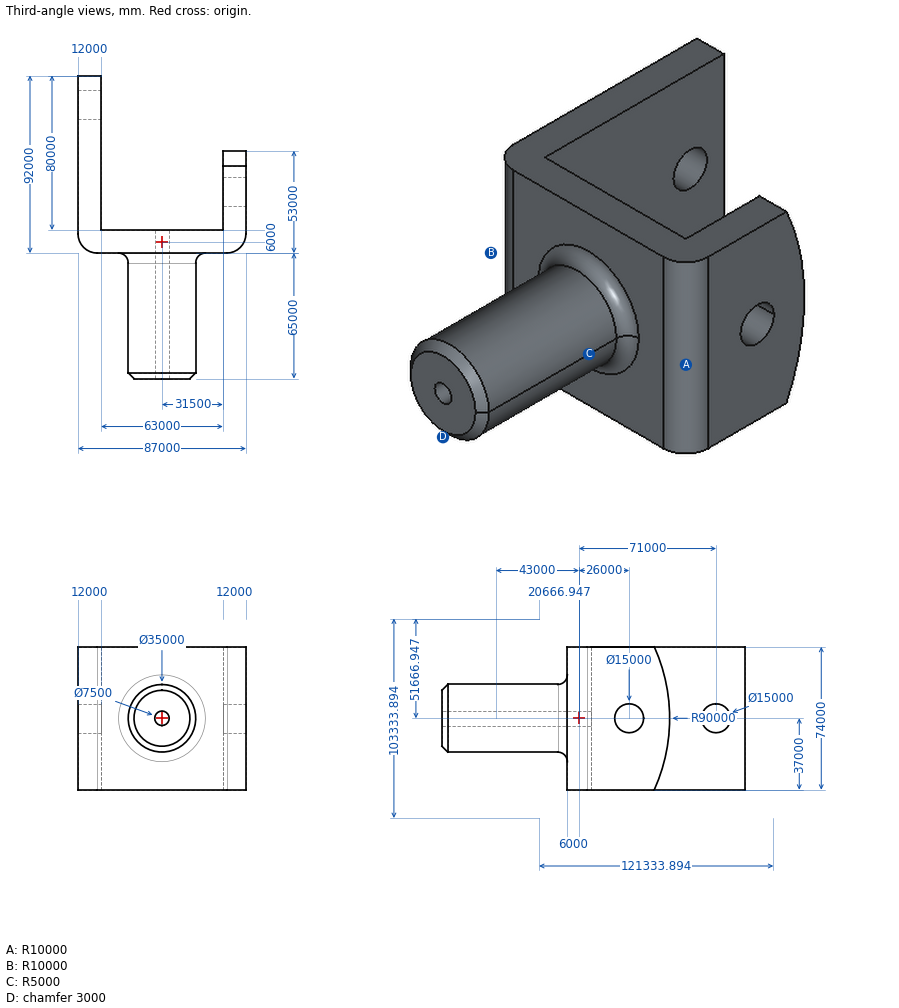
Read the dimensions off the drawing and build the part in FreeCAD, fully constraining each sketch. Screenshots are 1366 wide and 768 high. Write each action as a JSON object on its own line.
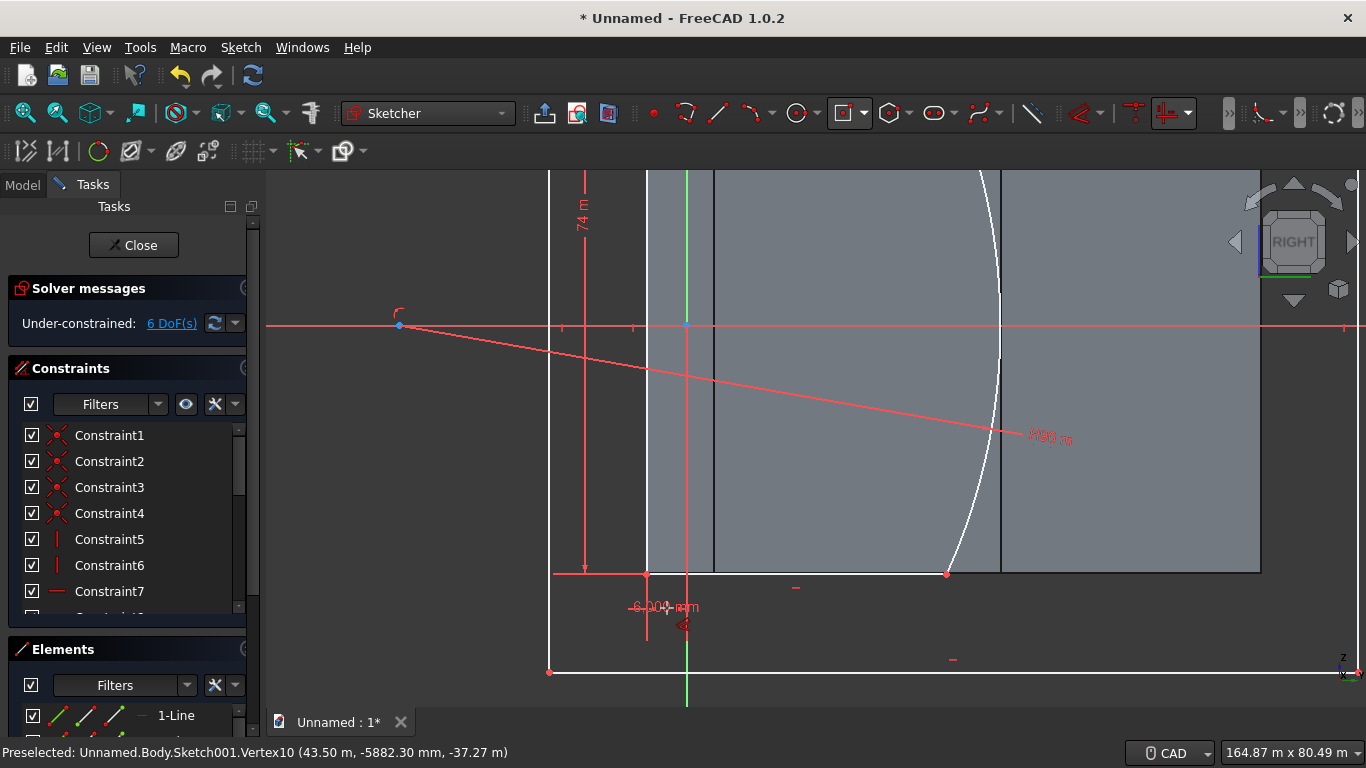
{"action": "left_click", "coordinate": [947, 574]}
{"action": "left_click", "coordinate": [981, 393]}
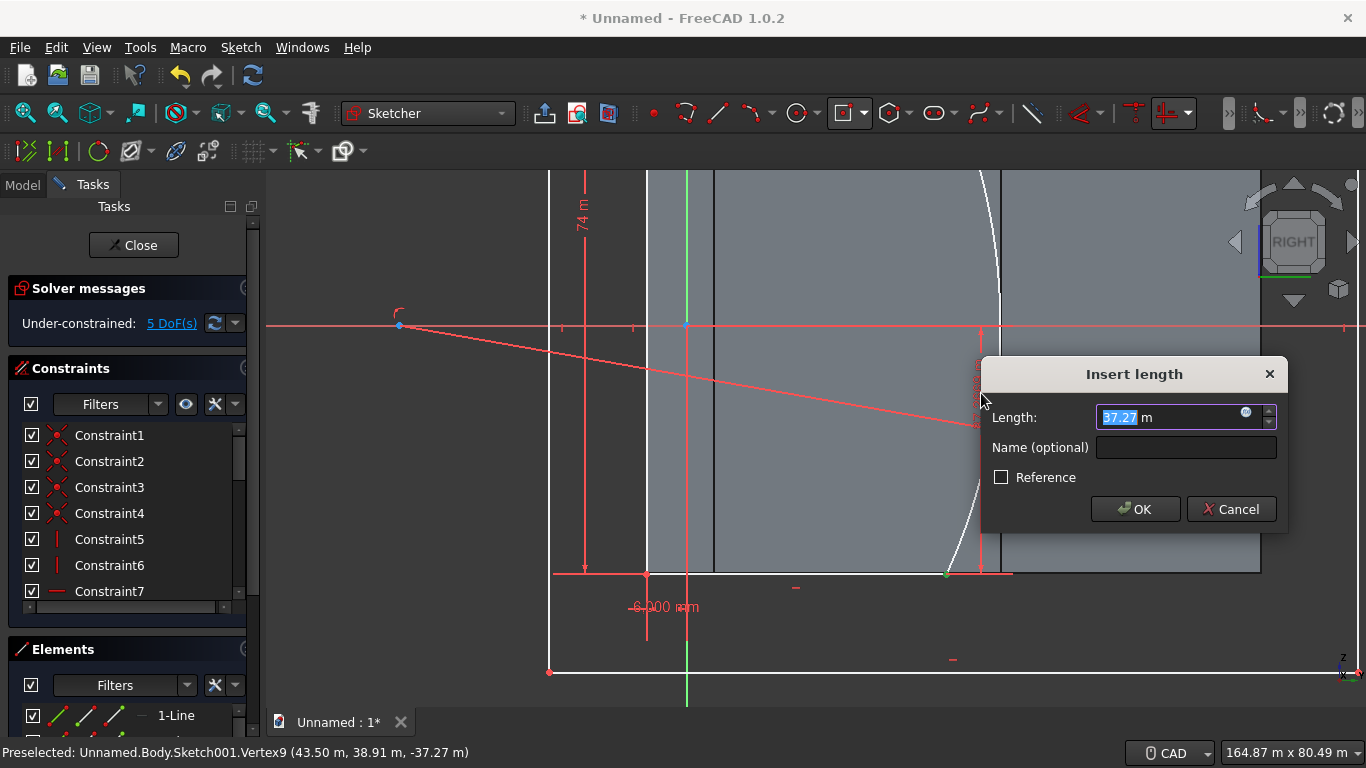
{"action": "key", "text": "ctrl+a"}
{"action": "type", "text": "37000 mm"}
{"action": "key", "text": "Return"}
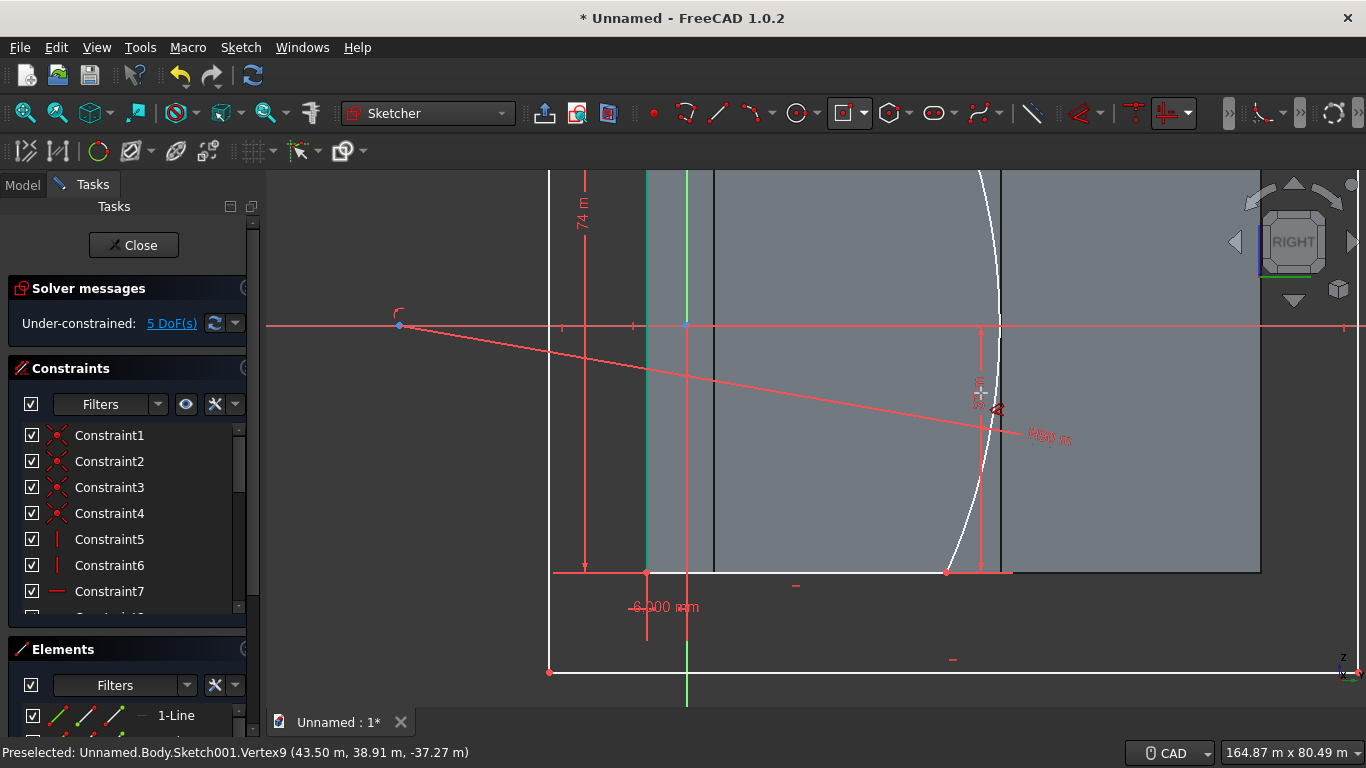
{"action": "left_click", "coordinate": [399, 326]}
{"action": "left_click", "coordinate": [477, 360]}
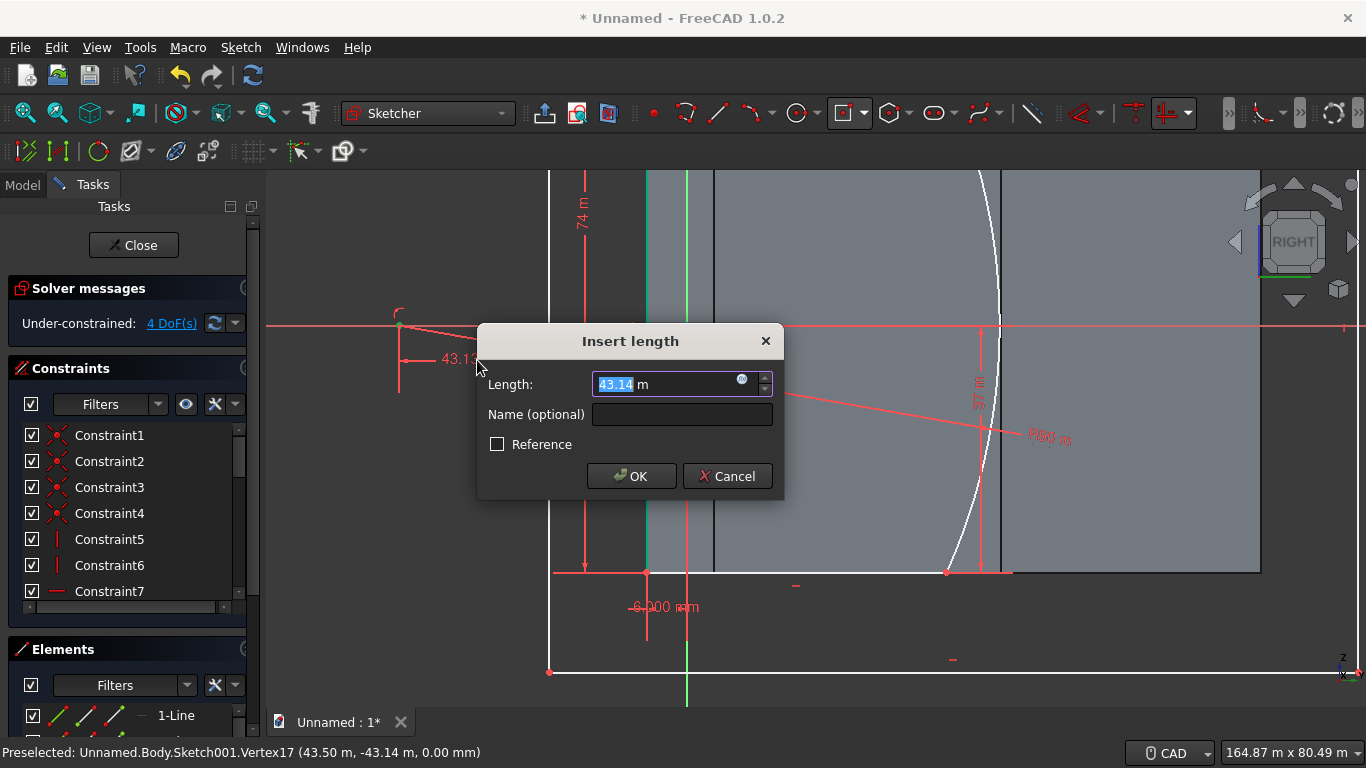
{"action": "key", "text": "ctrl+a"}
{"action": "type", "text": "43000 mm"}
{"action": "key", "text": "Return"}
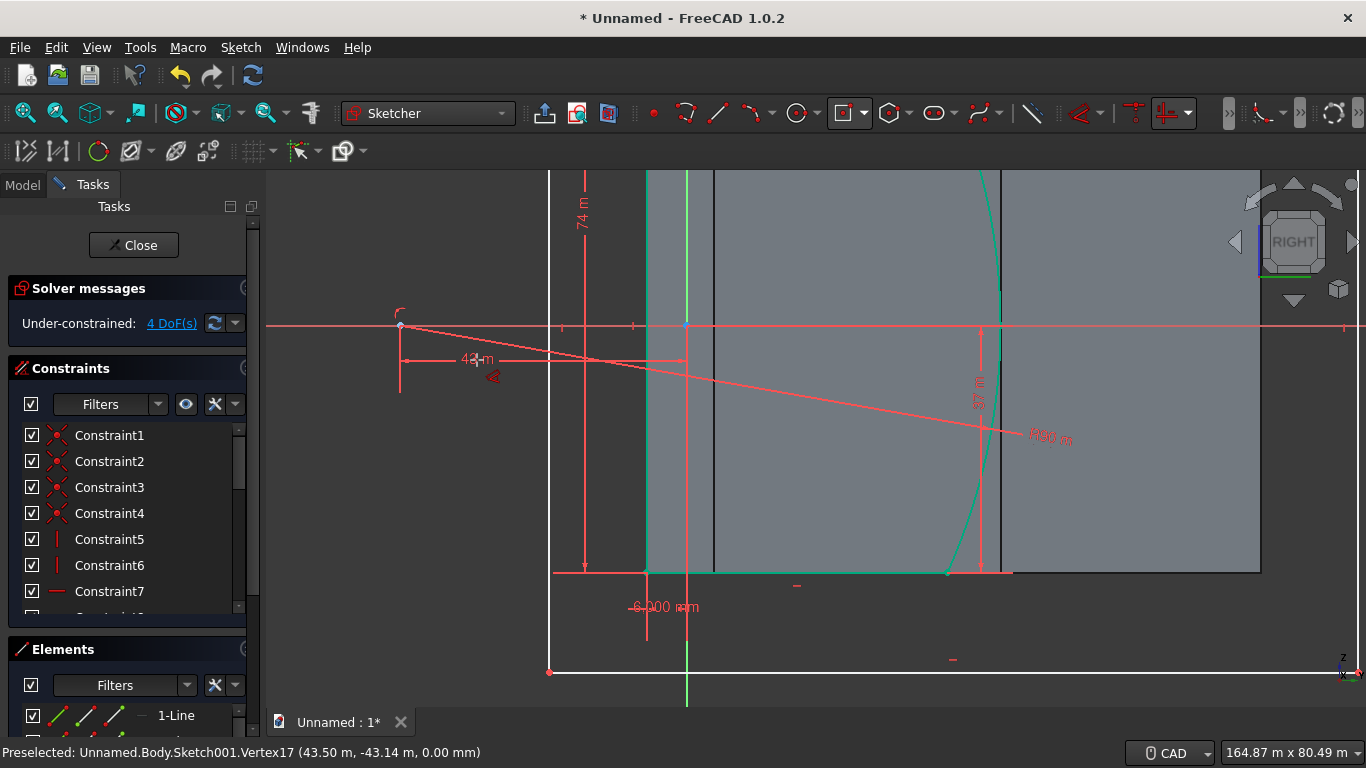
{"action": "left_click", "coordinate": [549, 466]}
{"action": "left_click", "coordinate": [515, 435]}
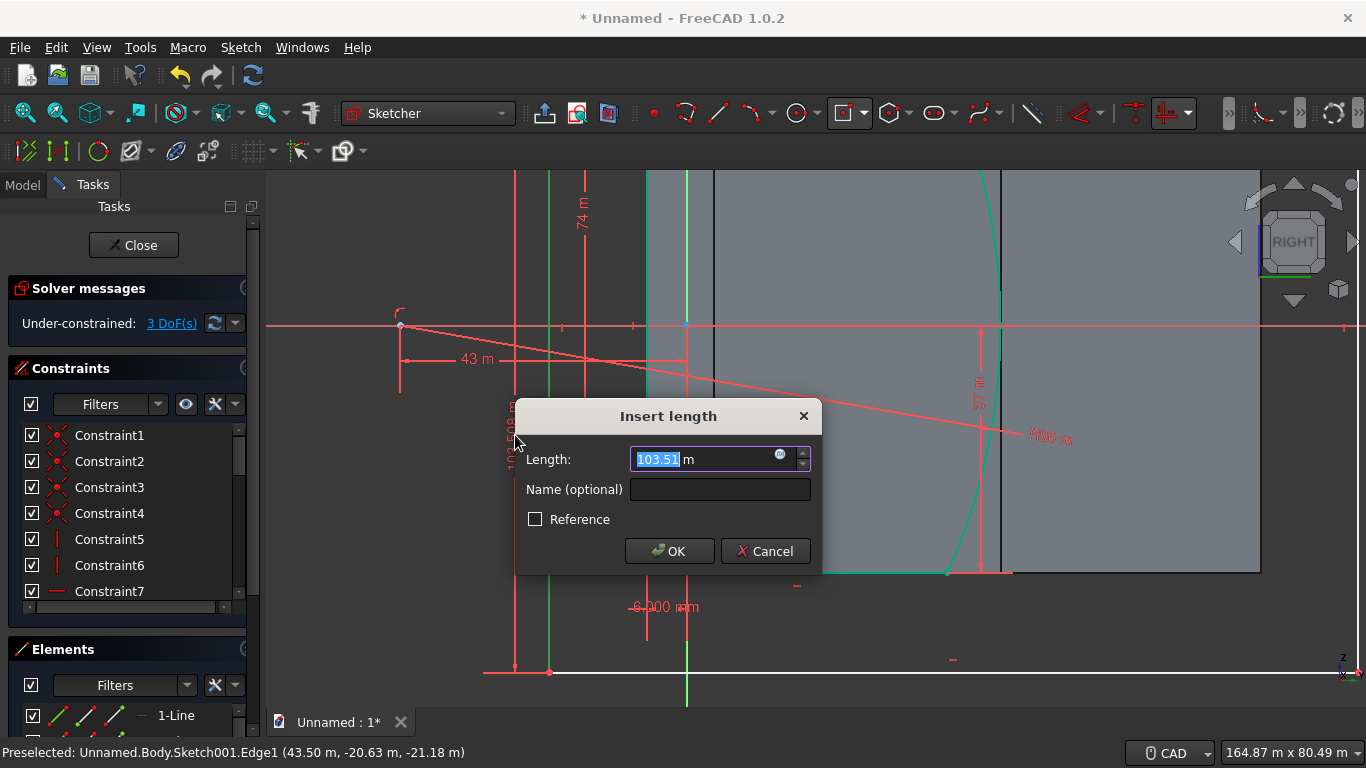
{"action": "key", "text": "ctrl+a"}
{"action": "type", "text": "103333.894 mm"}
{"action": "key", "text": "Return"}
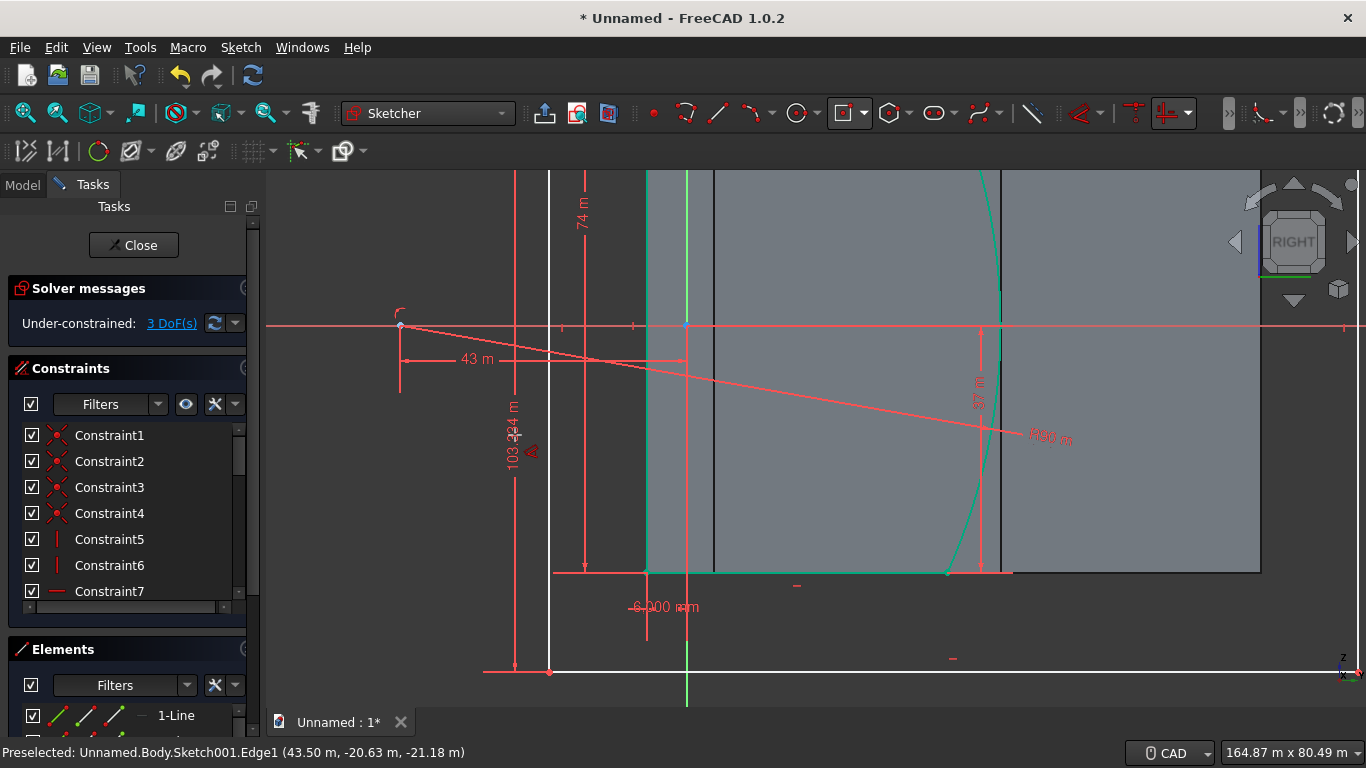
{"action": "left_click", "coordinate": [792, 672]}
{"action": "left_click", "coordinate": [875, 638]}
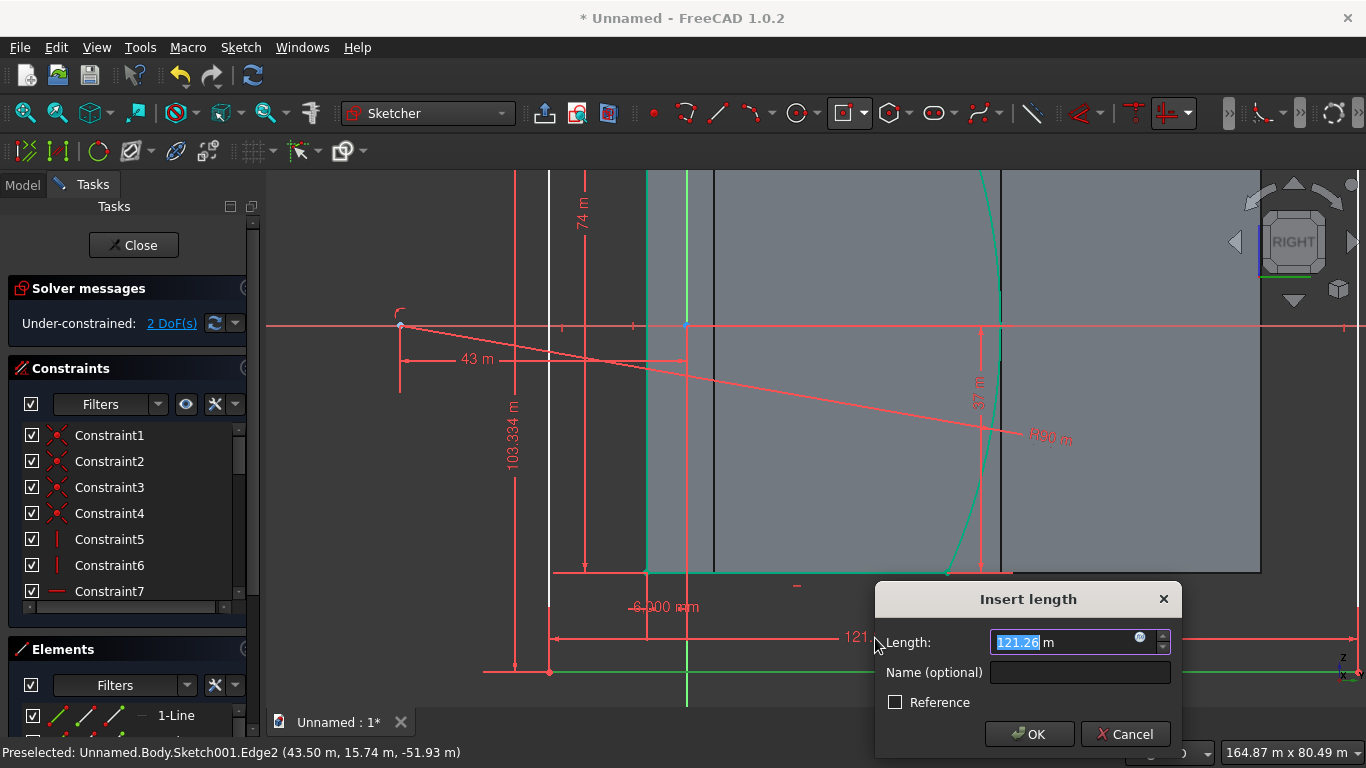
{"action": "key", "text": "ctrl+a"}
{"action": "type", "text": "121333.894 mm"}
{"action": "key", "text": "Return"}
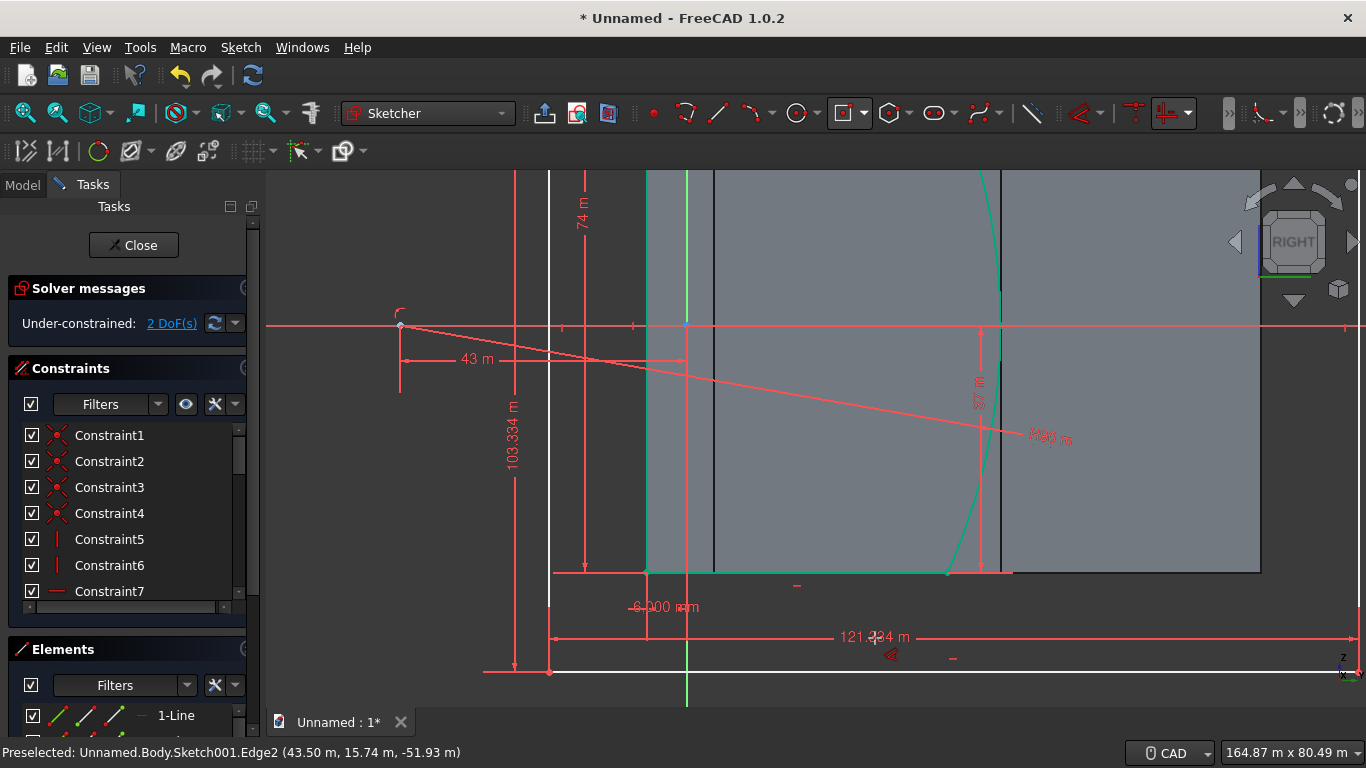
{"action": "scroll", "coordinate": [579, 531], "scroll_direction": "down", "scroll_amount": 4}